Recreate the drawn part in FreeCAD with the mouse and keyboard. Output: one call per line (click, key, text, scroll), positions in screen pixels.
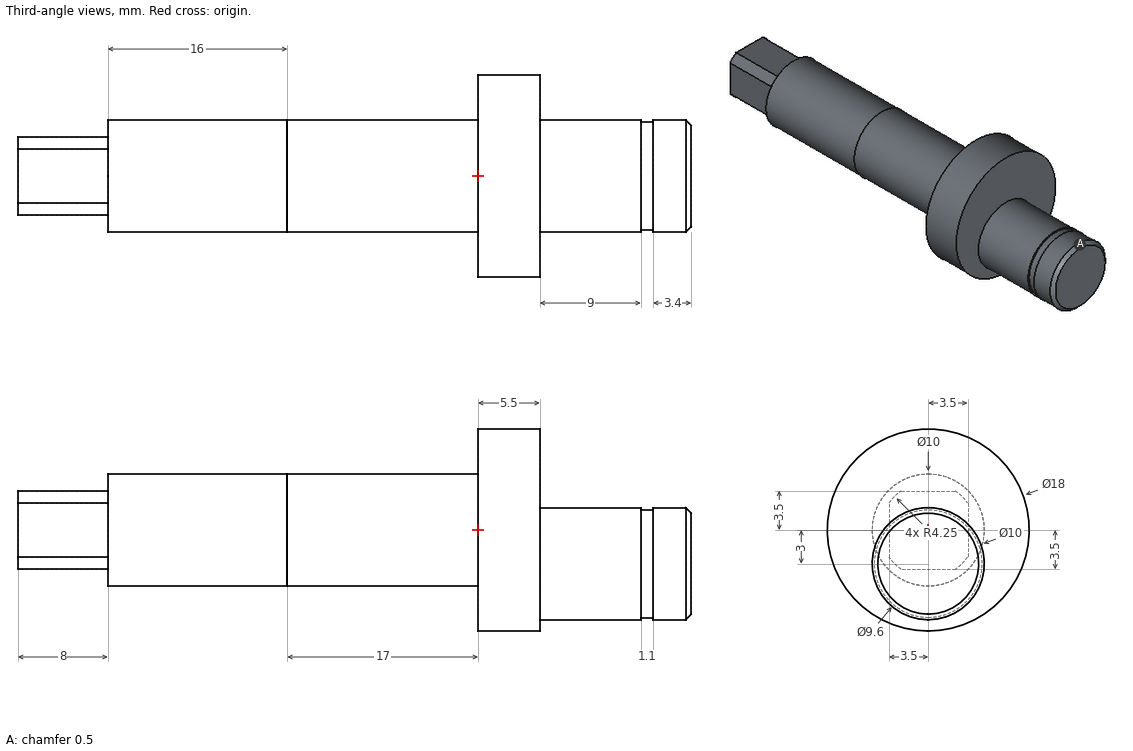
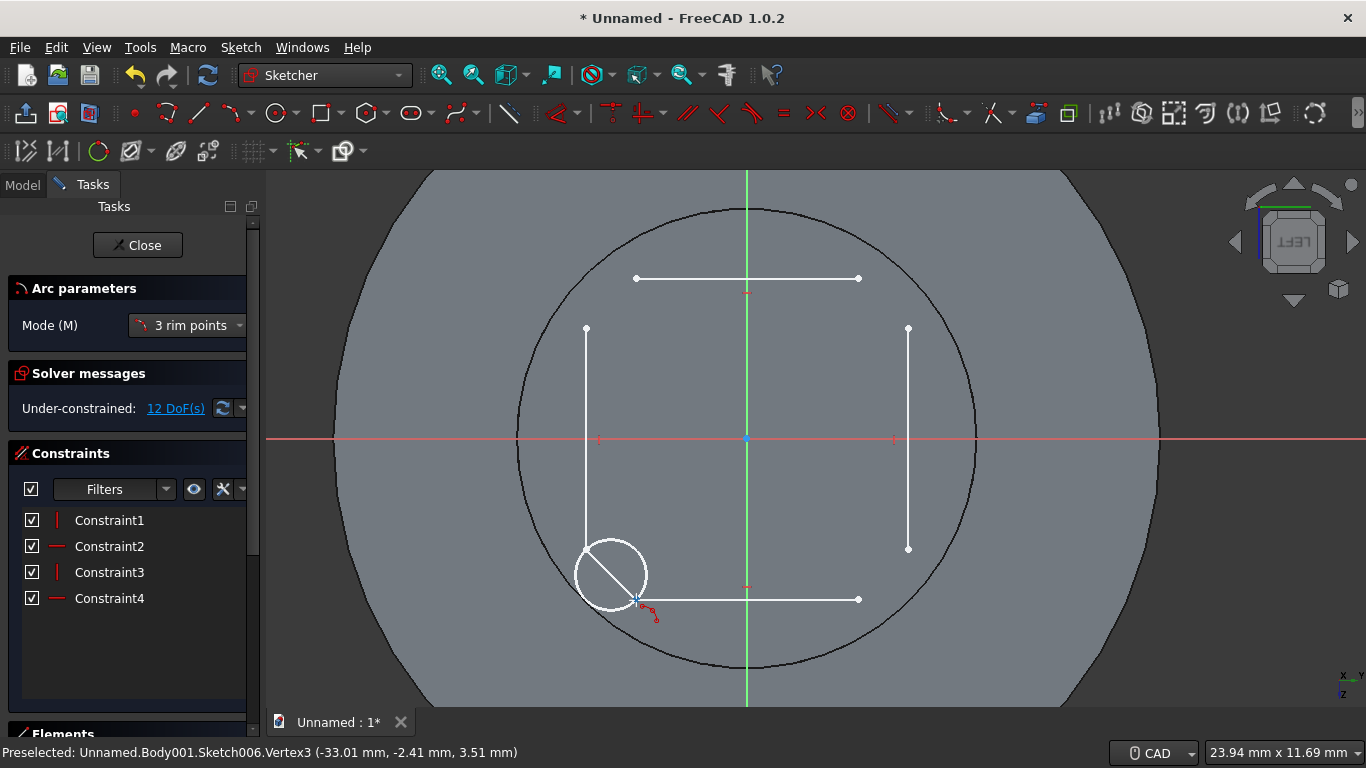
scroll(609, 577, up, 8)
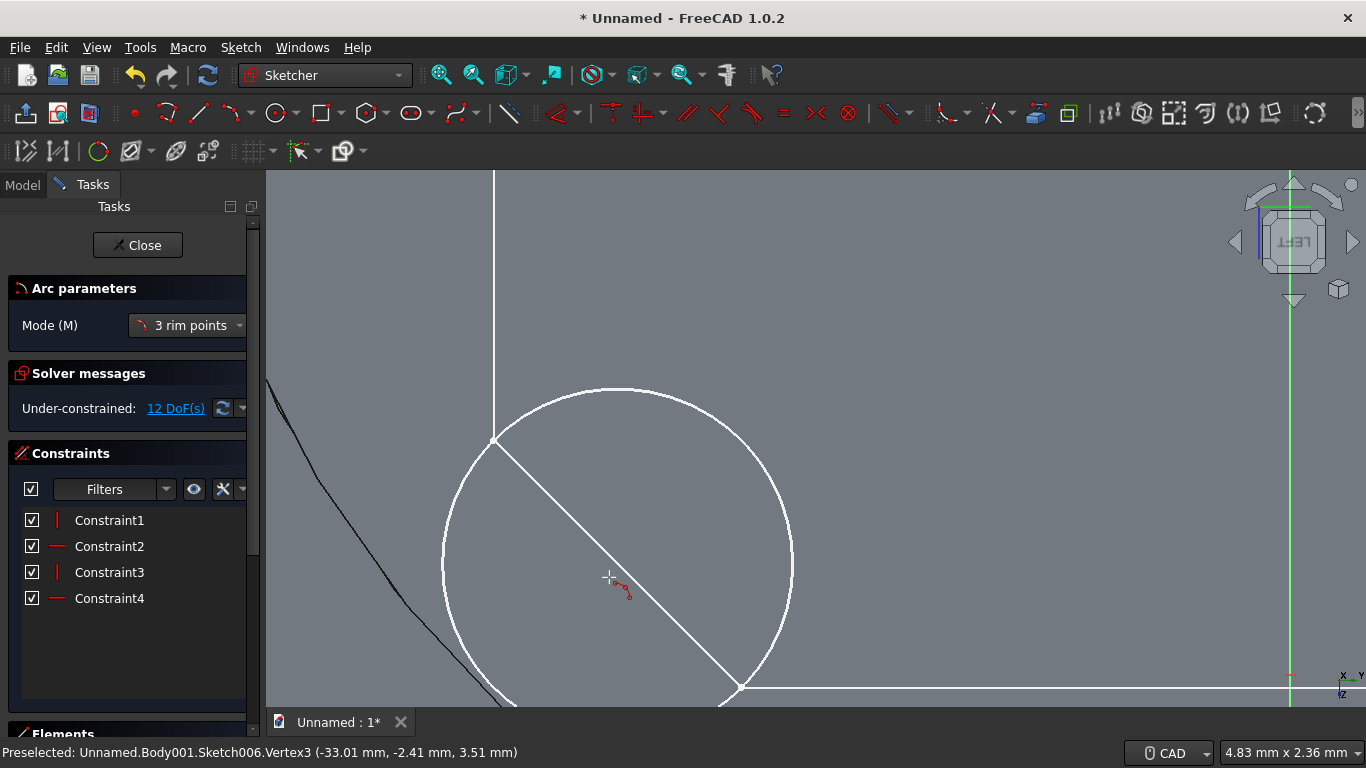
click(606, 572)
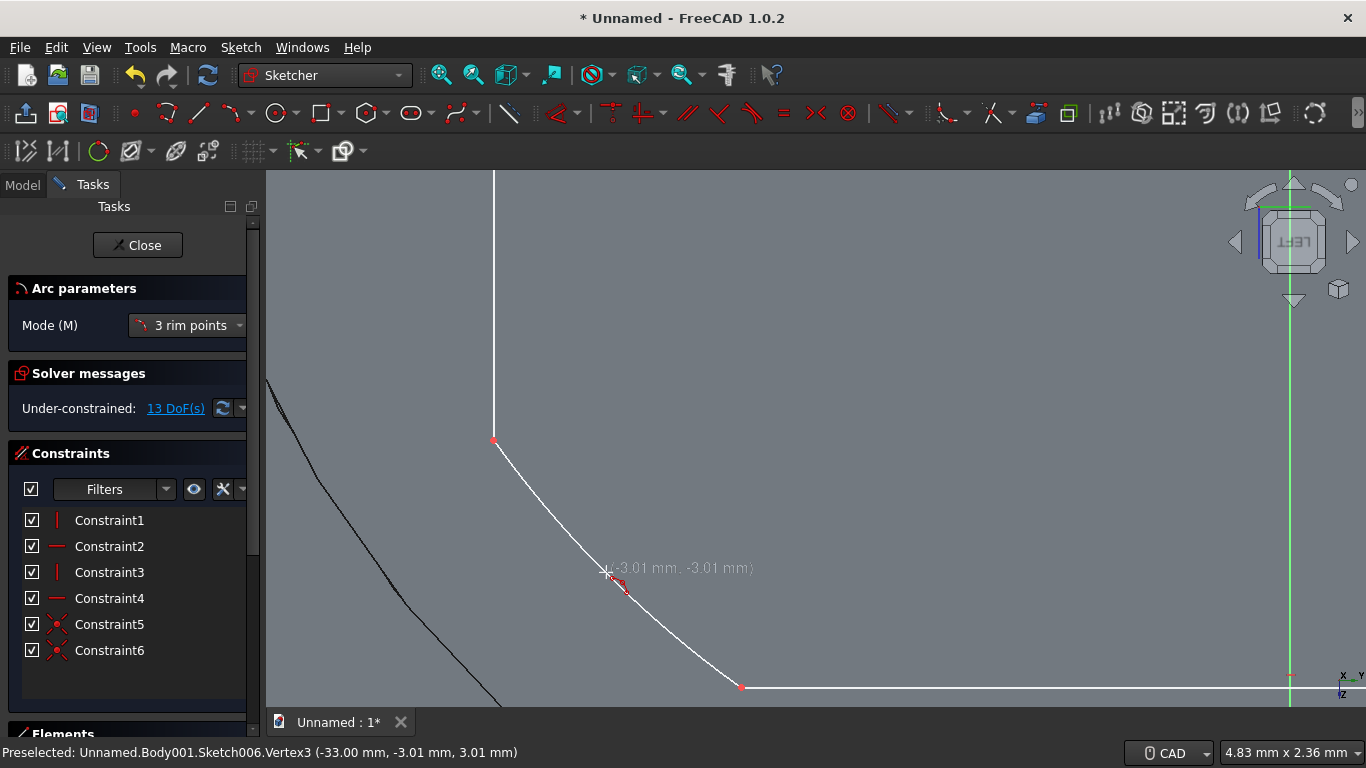
scroll(610, 578, down, 8)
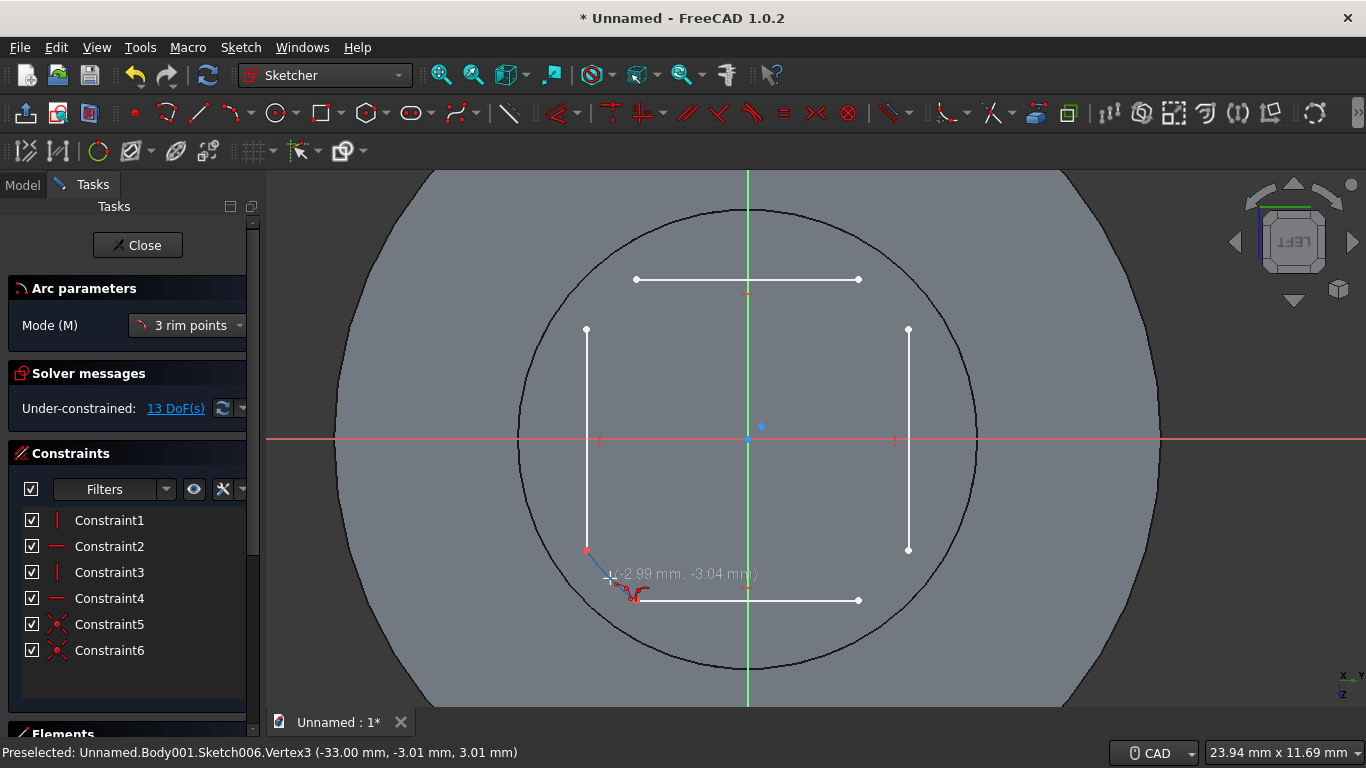
click(859, 601)
click(909, 551)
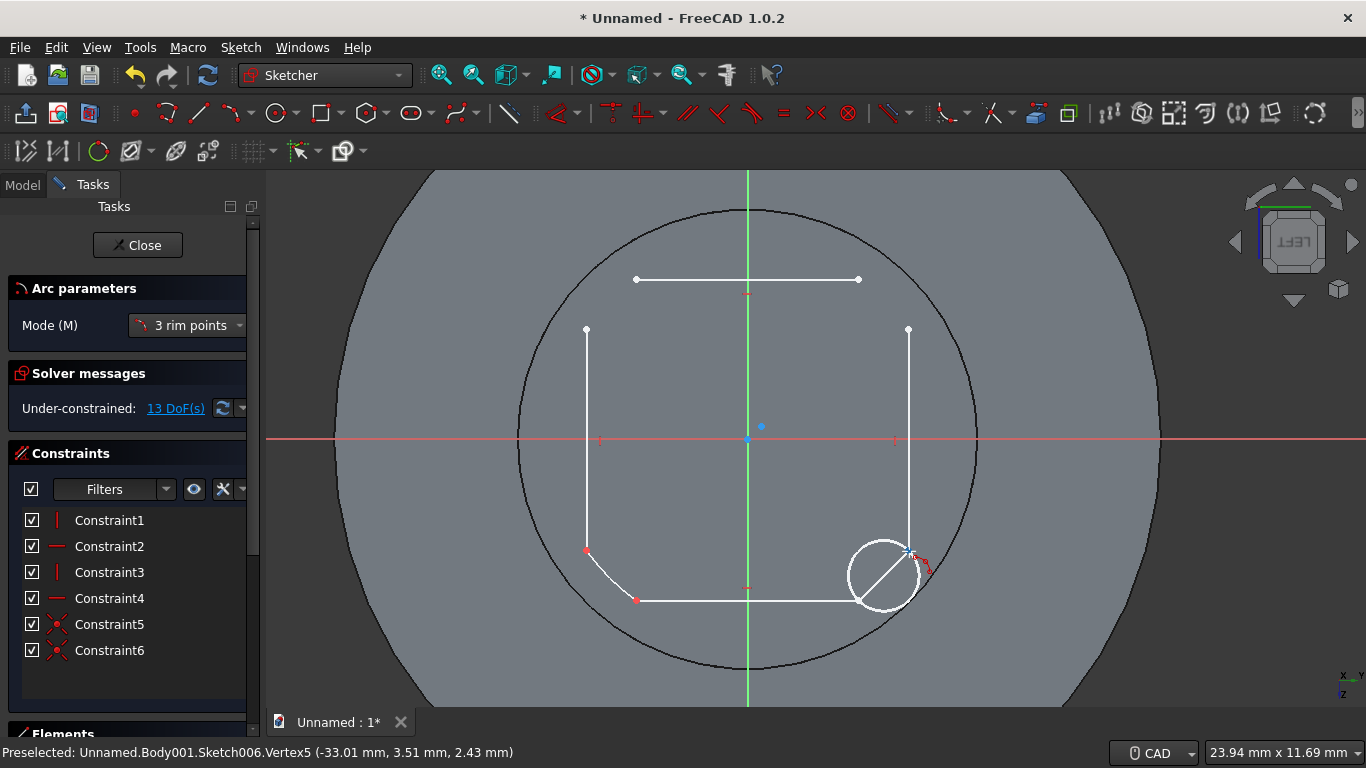
scroll(886, 577, up, 8)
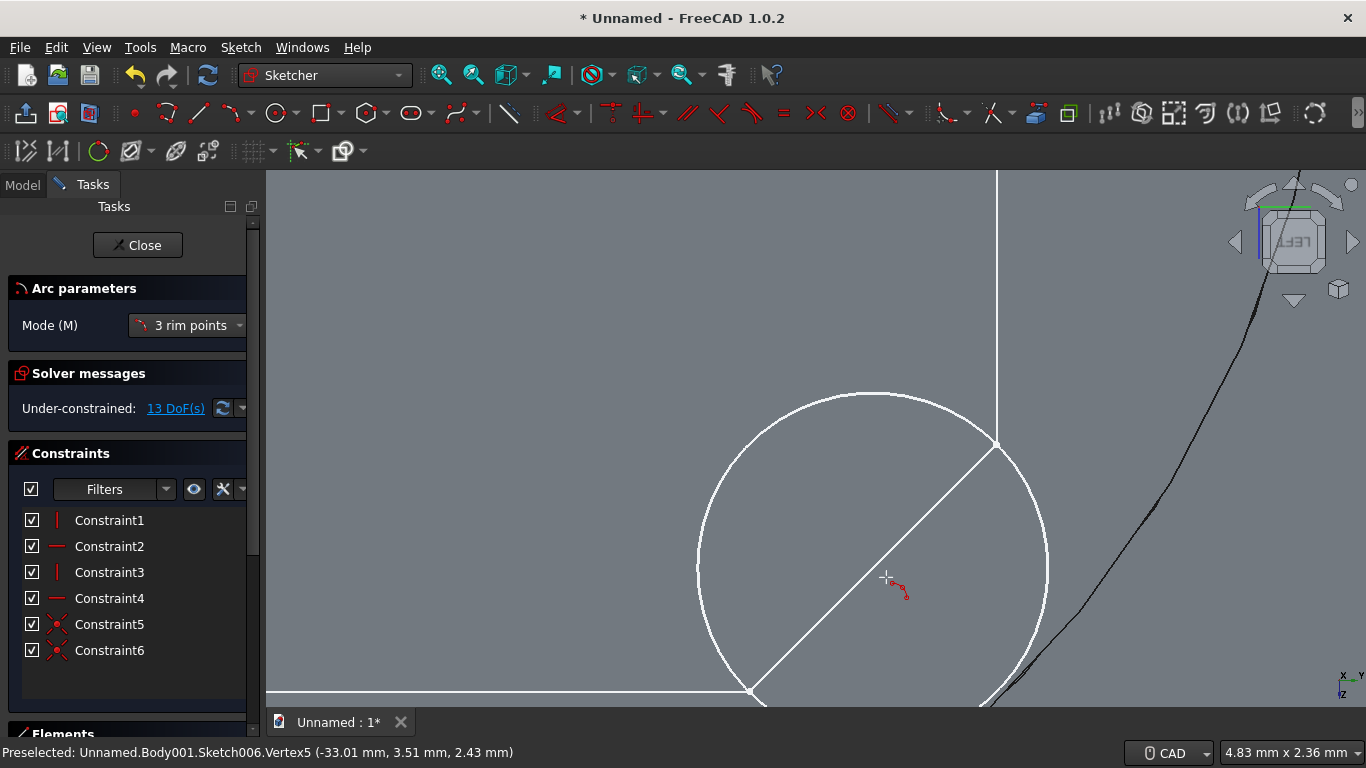
click(882, 576)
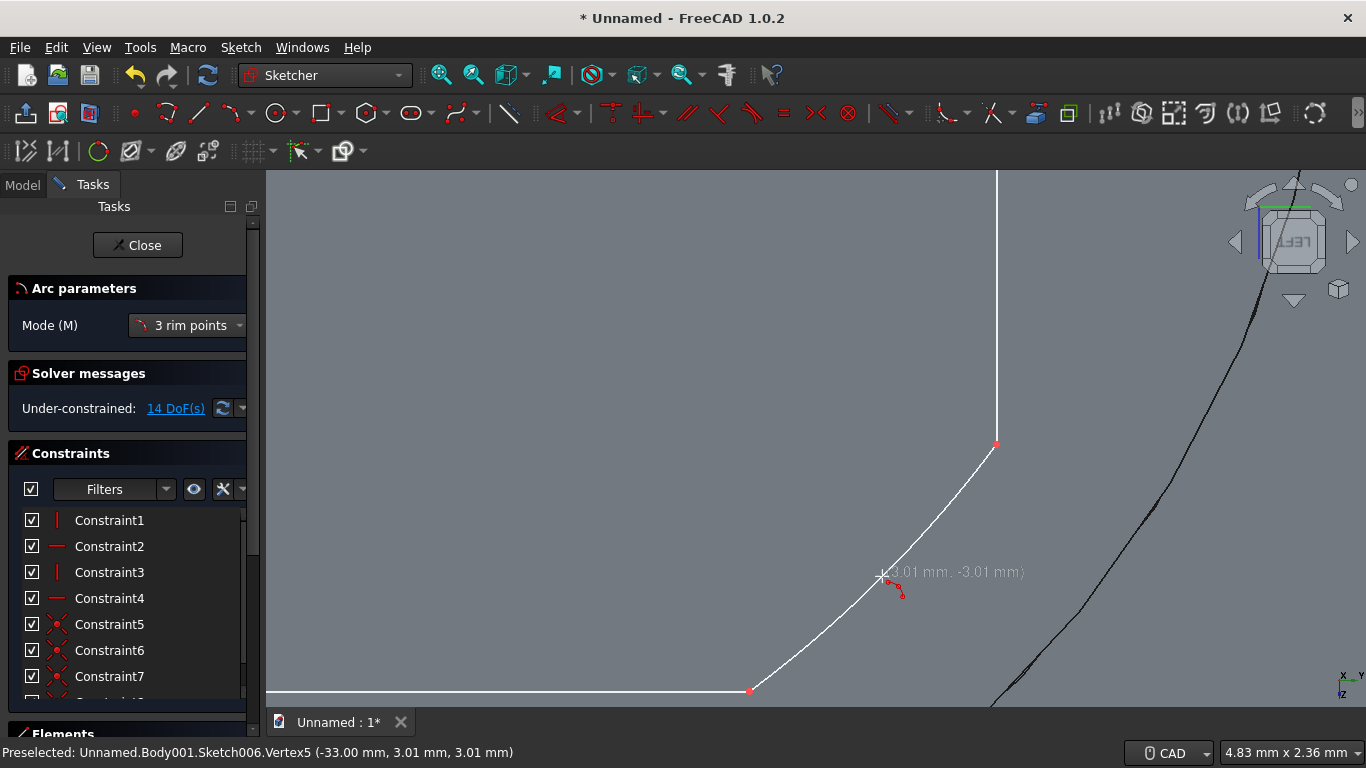
scroll(886, 577, down, 8)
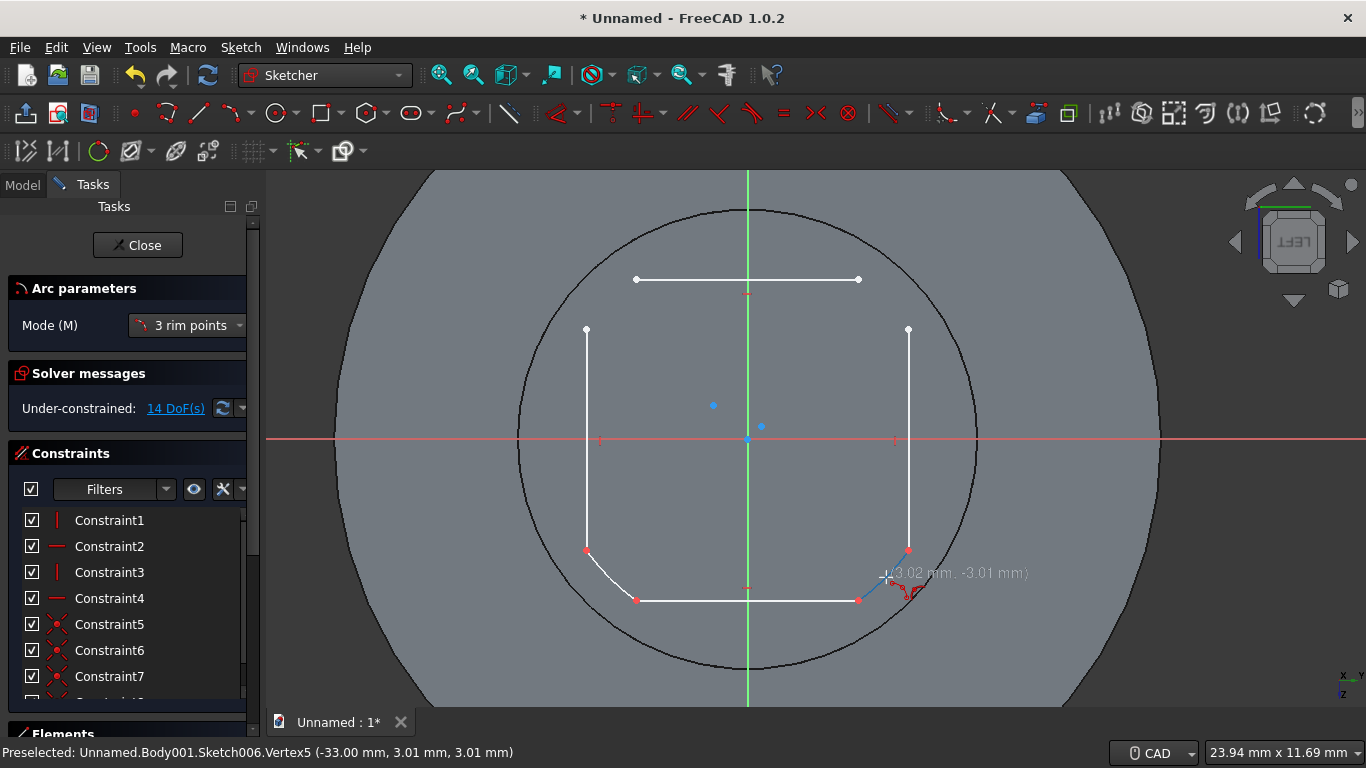
click(909, 330)
click(859, 280)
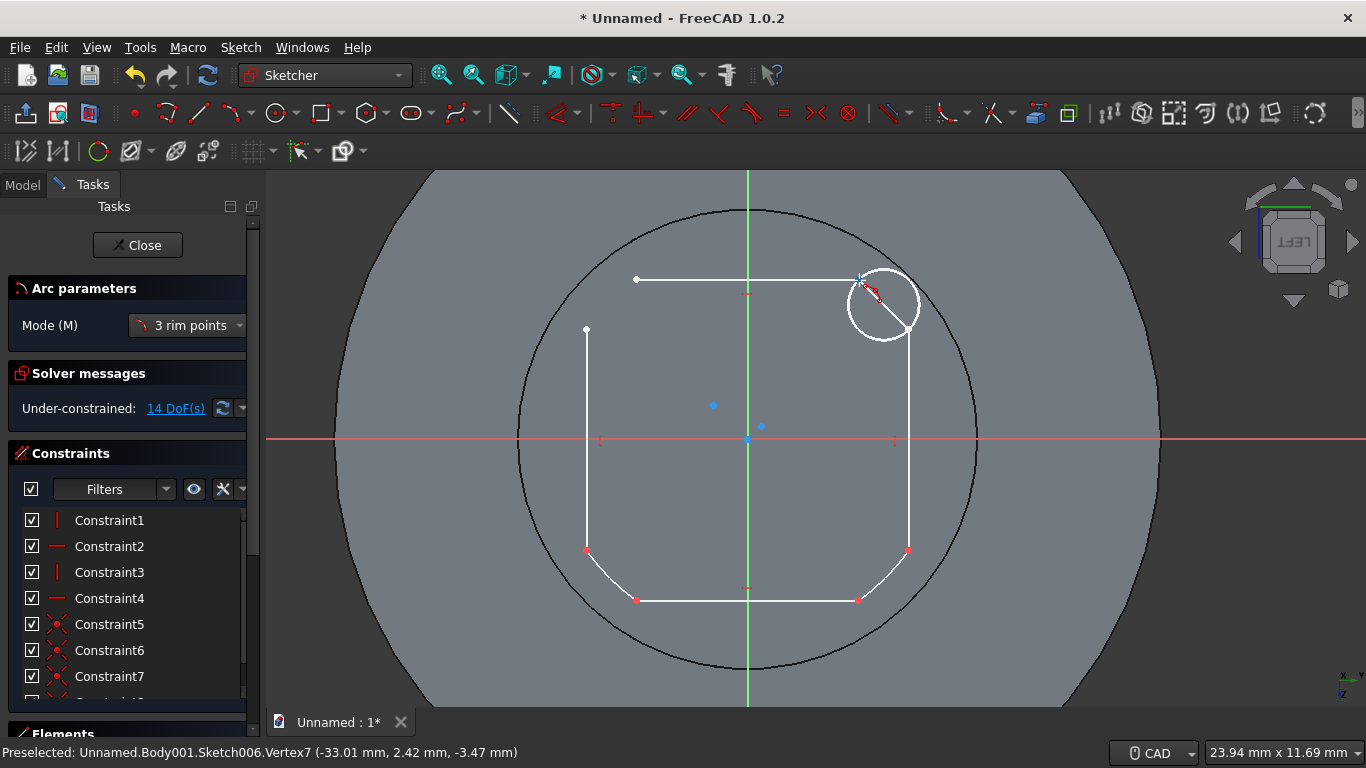
scroll(886, 301, up, 8)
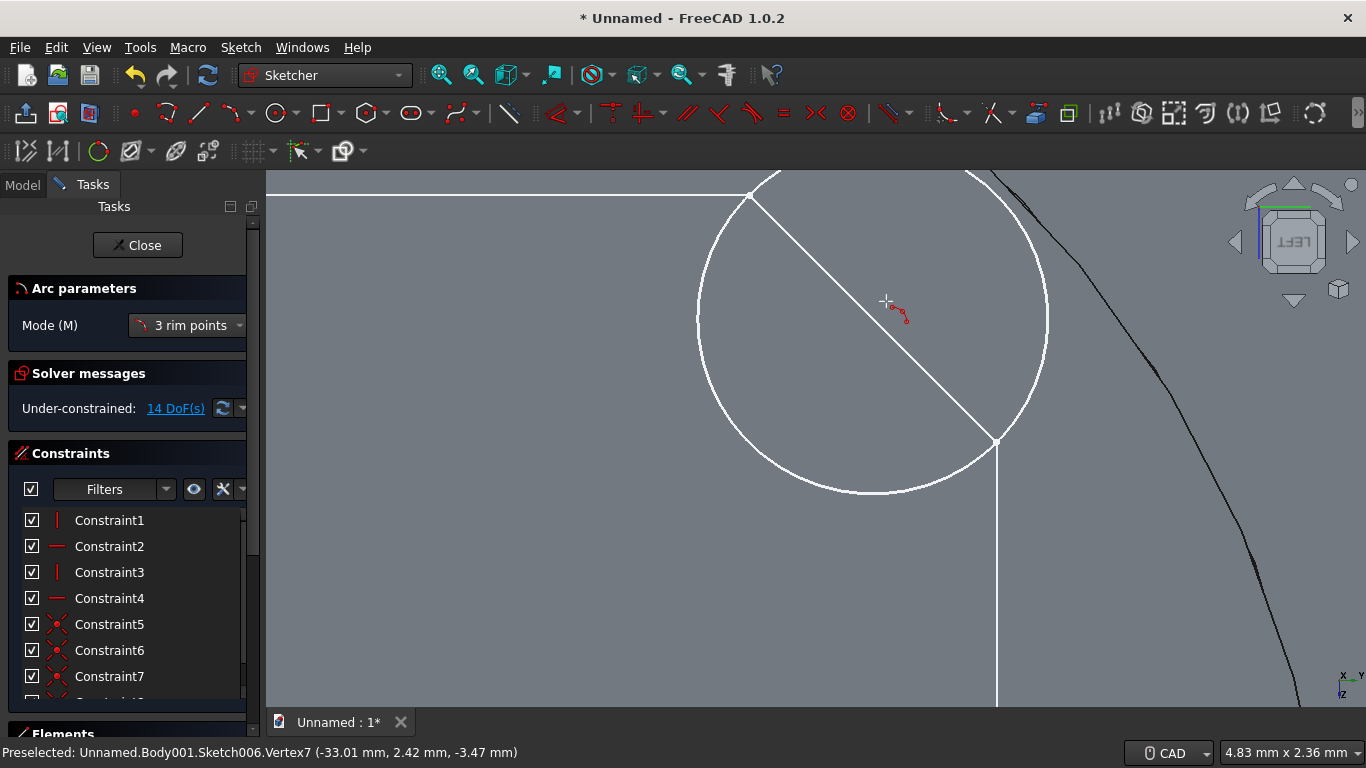
click(882, 301)